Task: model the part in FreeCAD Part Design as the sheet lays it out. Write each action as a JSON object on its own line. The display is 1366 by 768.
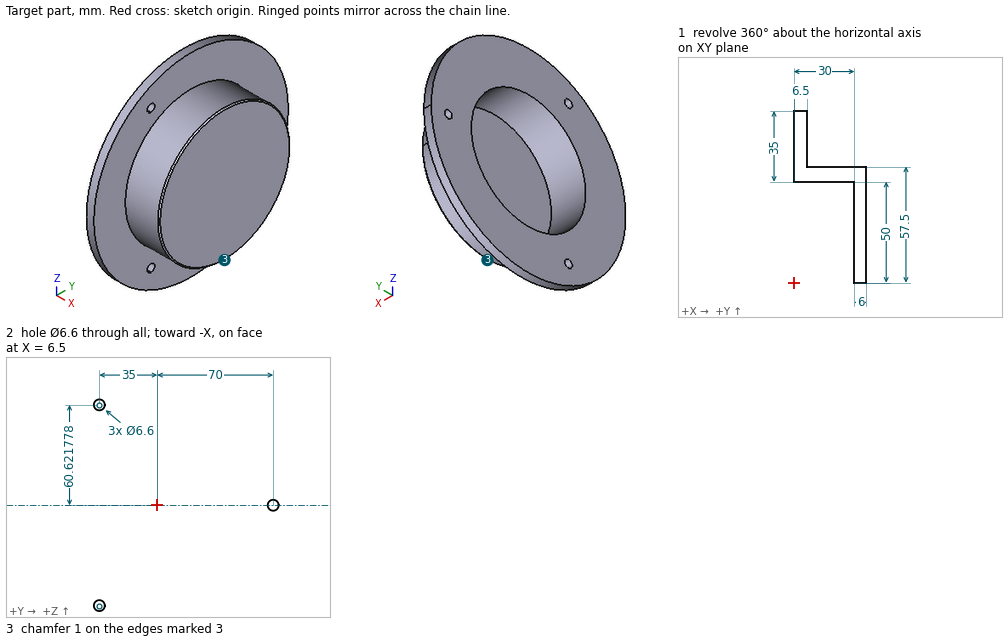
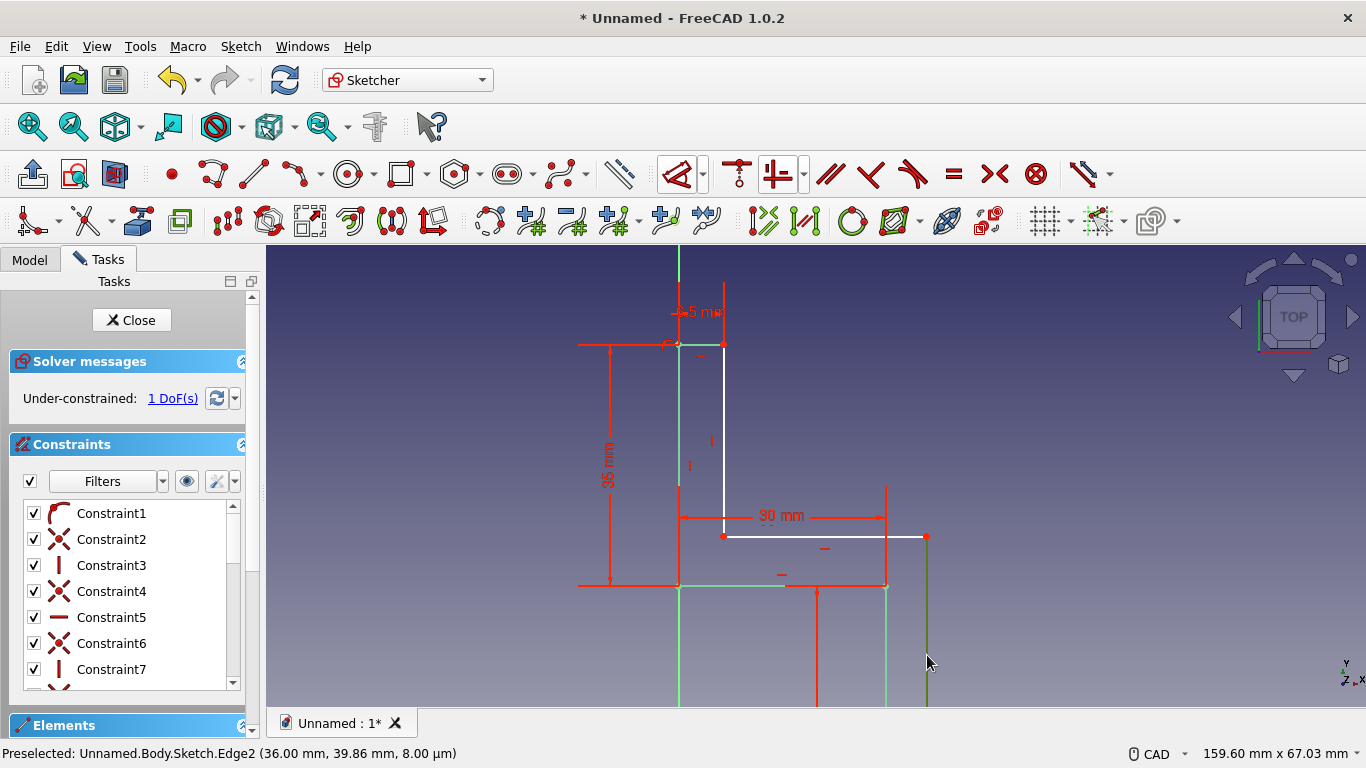
{"action": "key", "text": "i"}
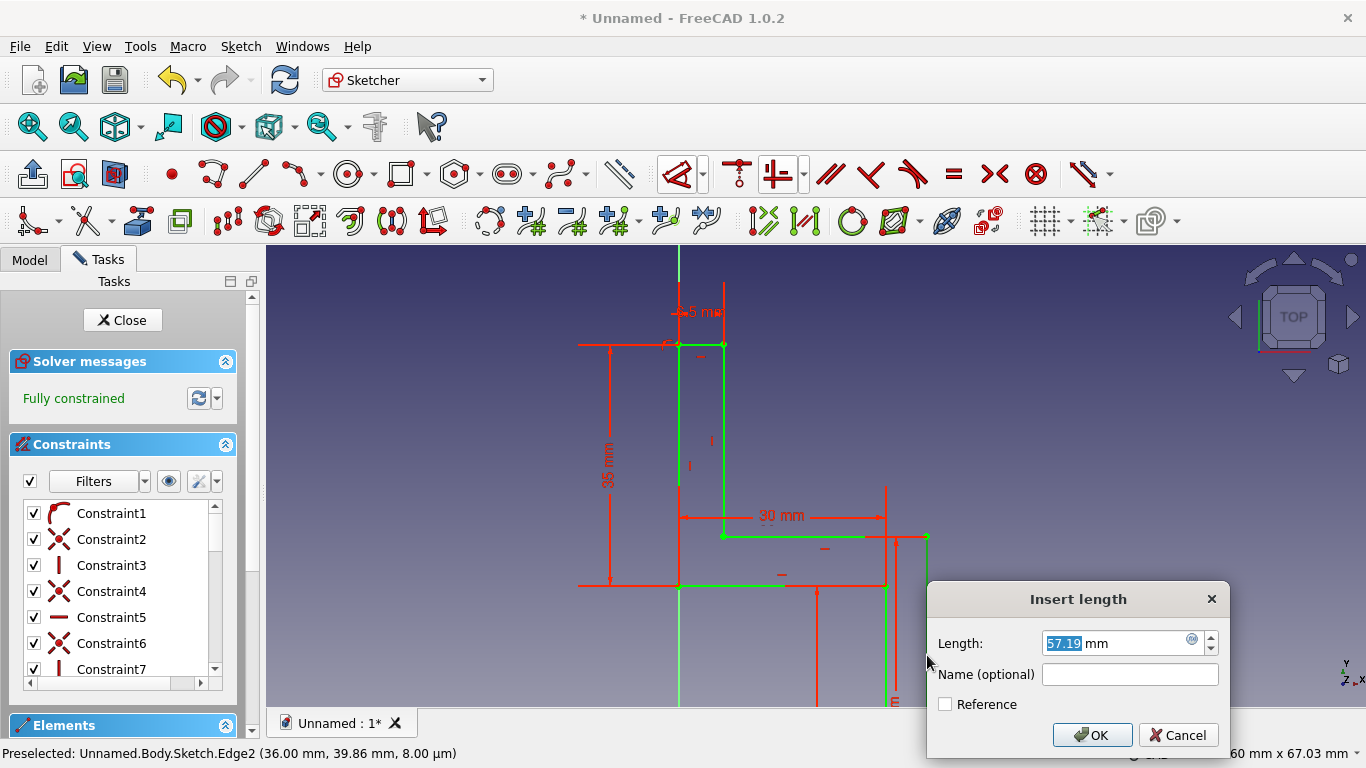
{"action": "type", "text": "57.5"}
{"action": "key", "text": "Return"}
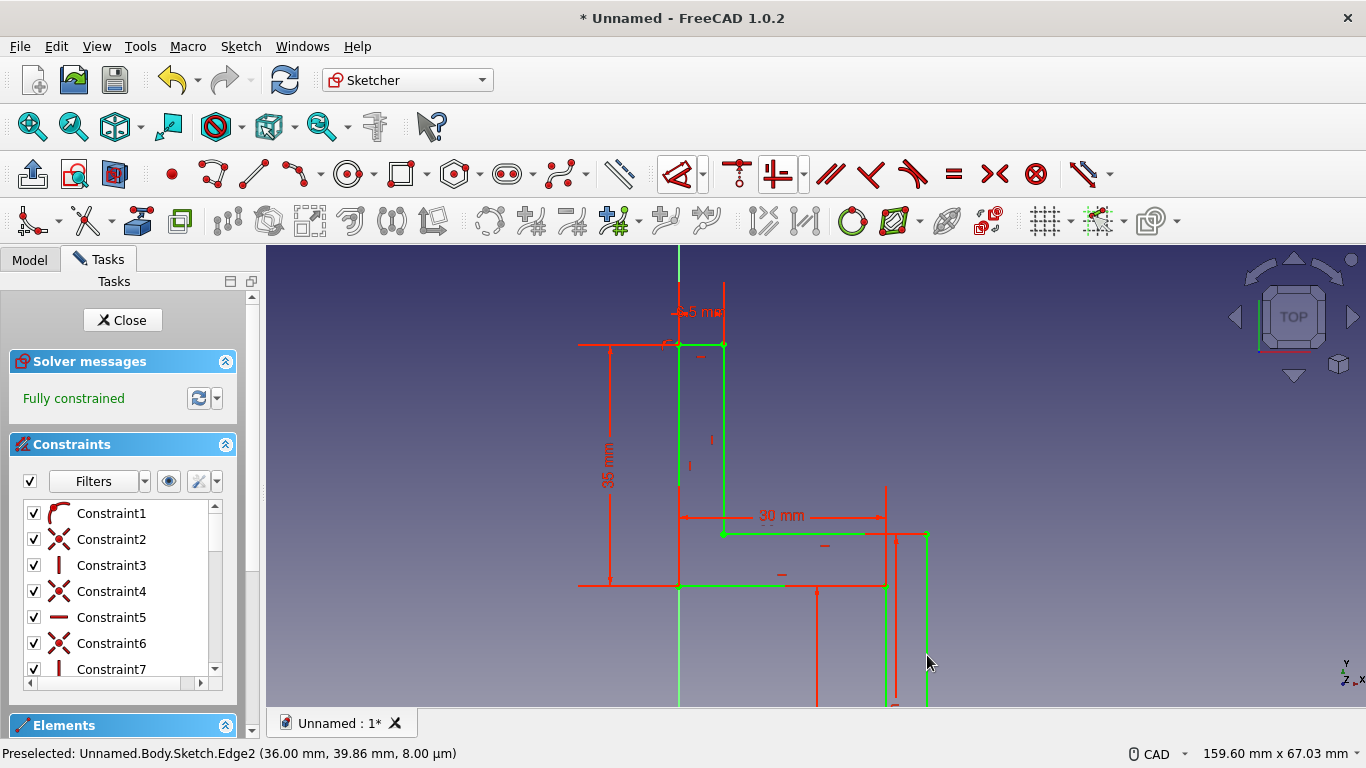
{"action": "left_click", "coordinate": [123, 320]}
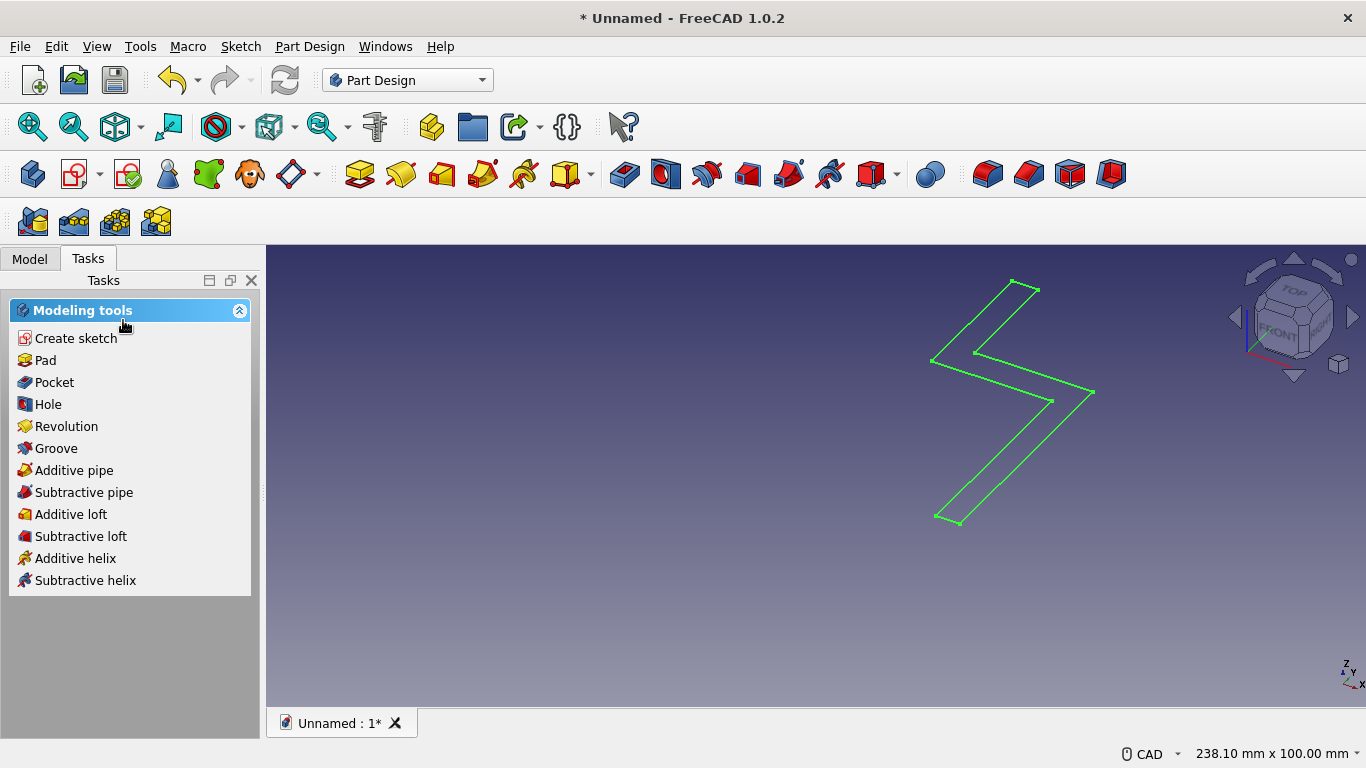
{"action": "left_click", "coordinate": [401, 174]}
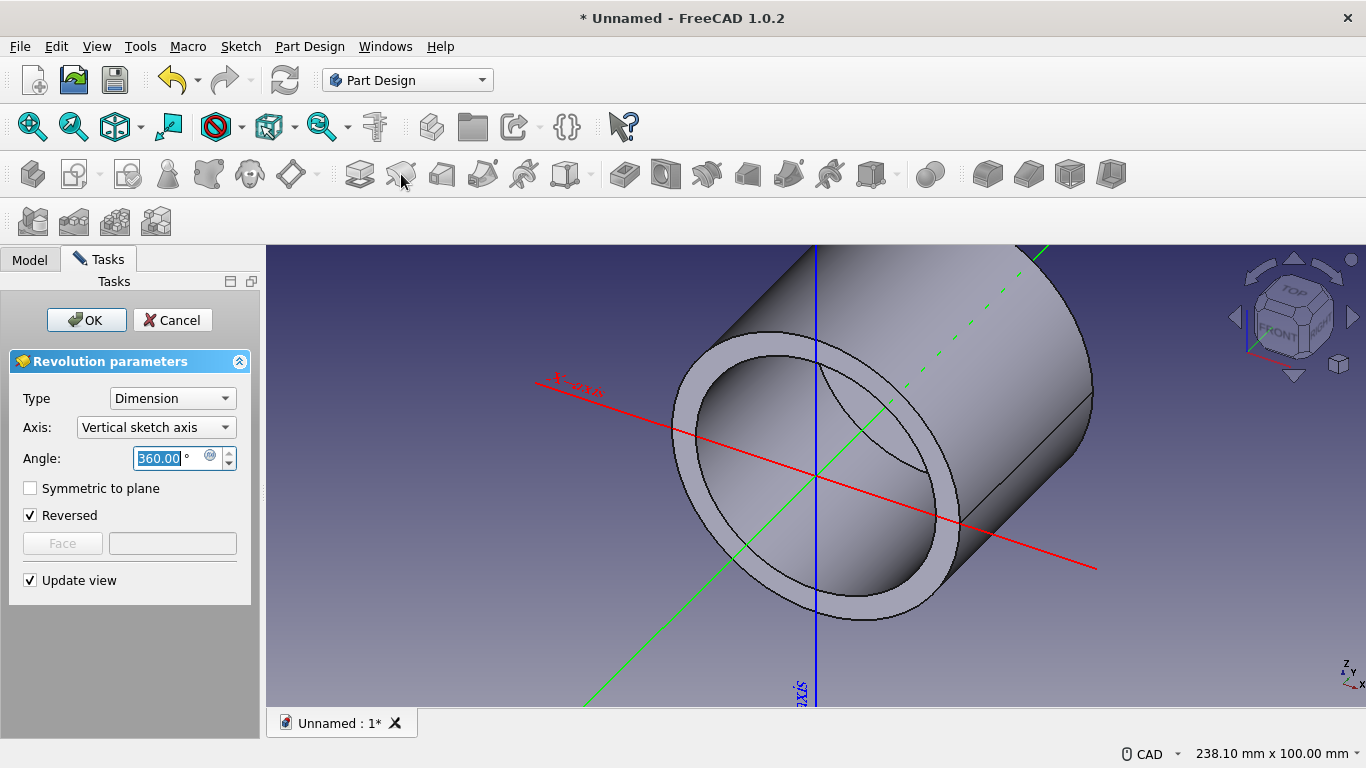
{"action": "left_click", "coordinate": [157, 428]}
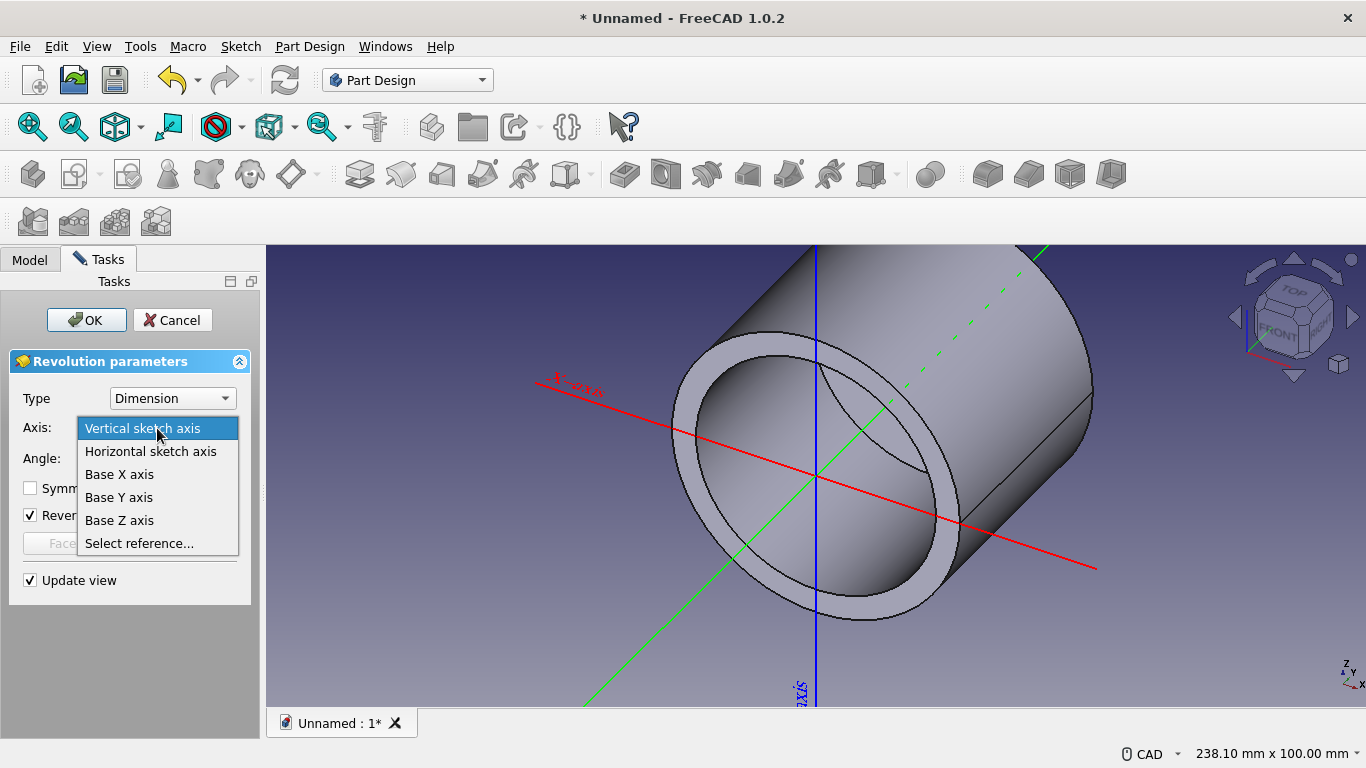
{"action": "left_click", "coordinate": [156, 452]}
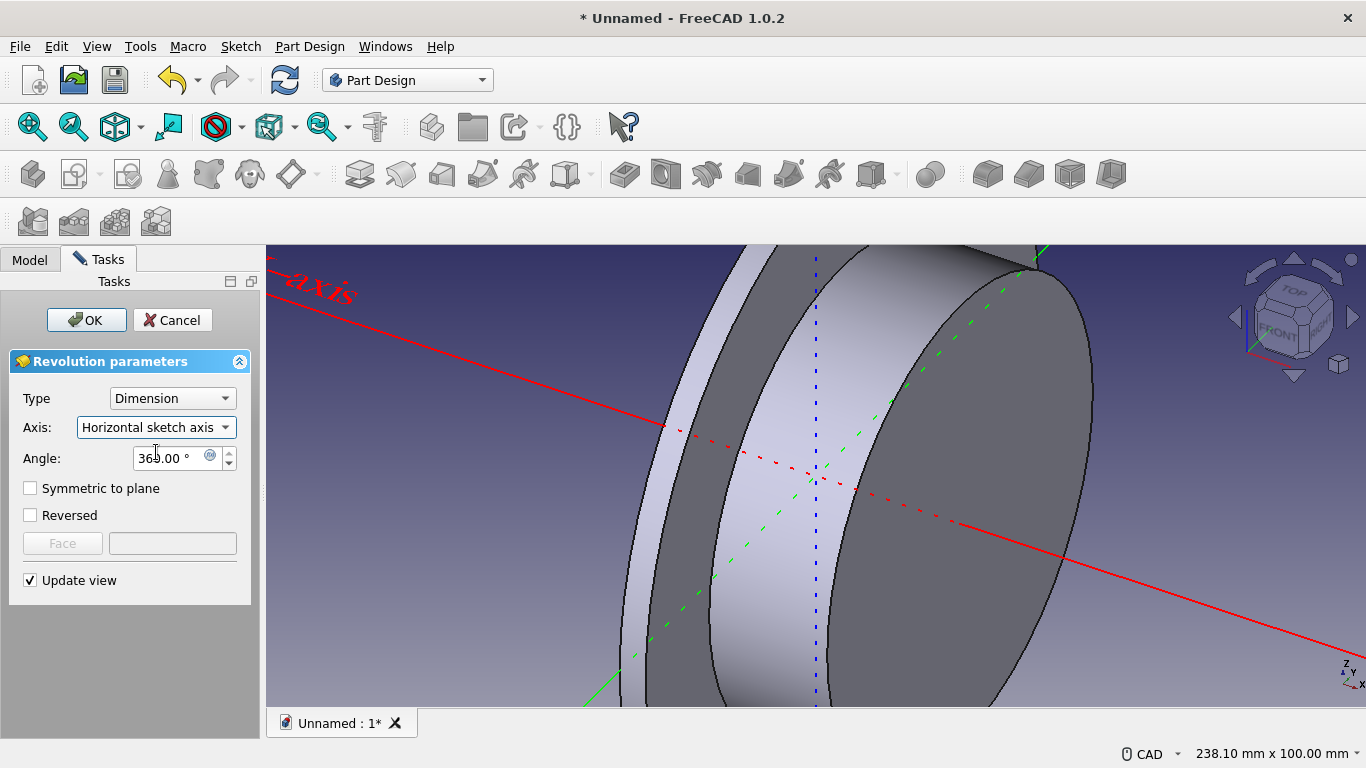
{"action": "left_click", "coordinate": [87, 320]}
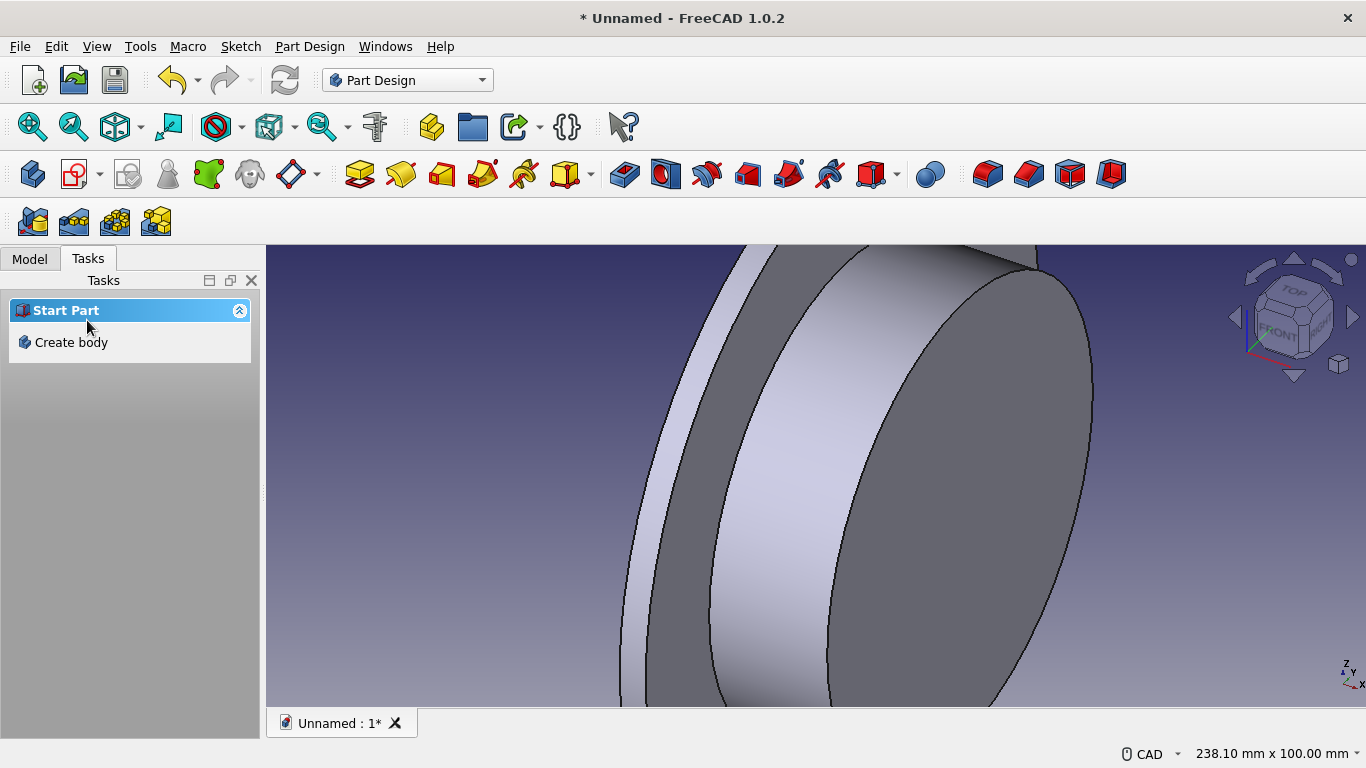
{"action": "left_click", "coordinate": [33, 128]}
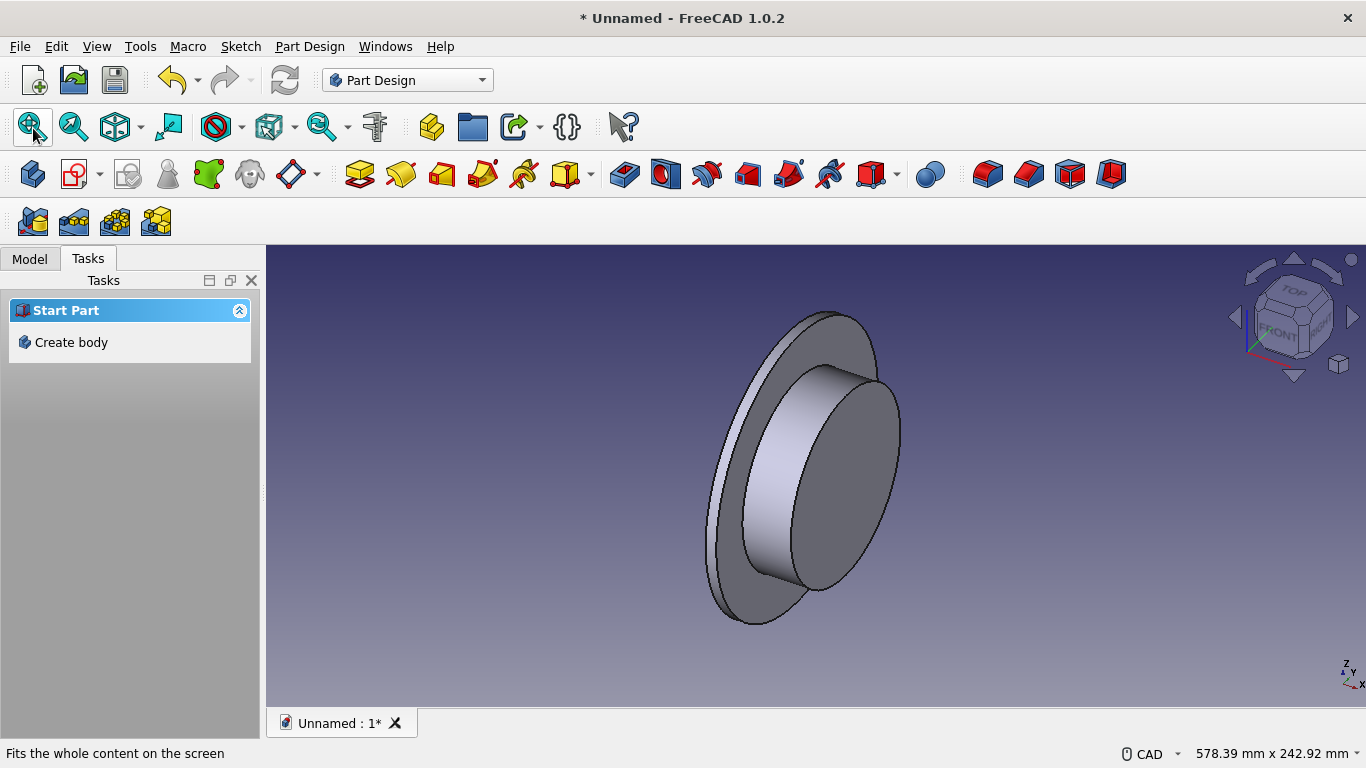
{"action": "left_click", "coordinate": [797, 355]}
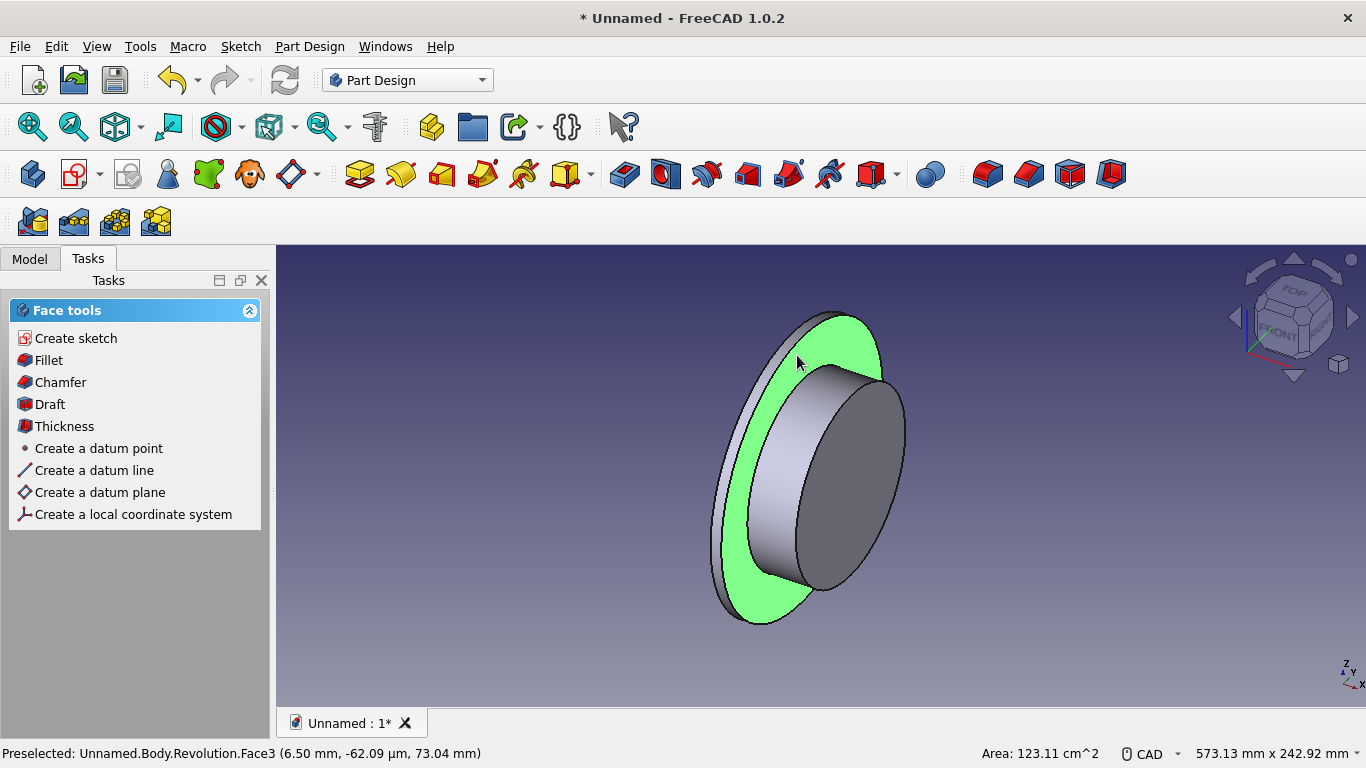
{"action": "left_click", "coordinate": [74, 174]}